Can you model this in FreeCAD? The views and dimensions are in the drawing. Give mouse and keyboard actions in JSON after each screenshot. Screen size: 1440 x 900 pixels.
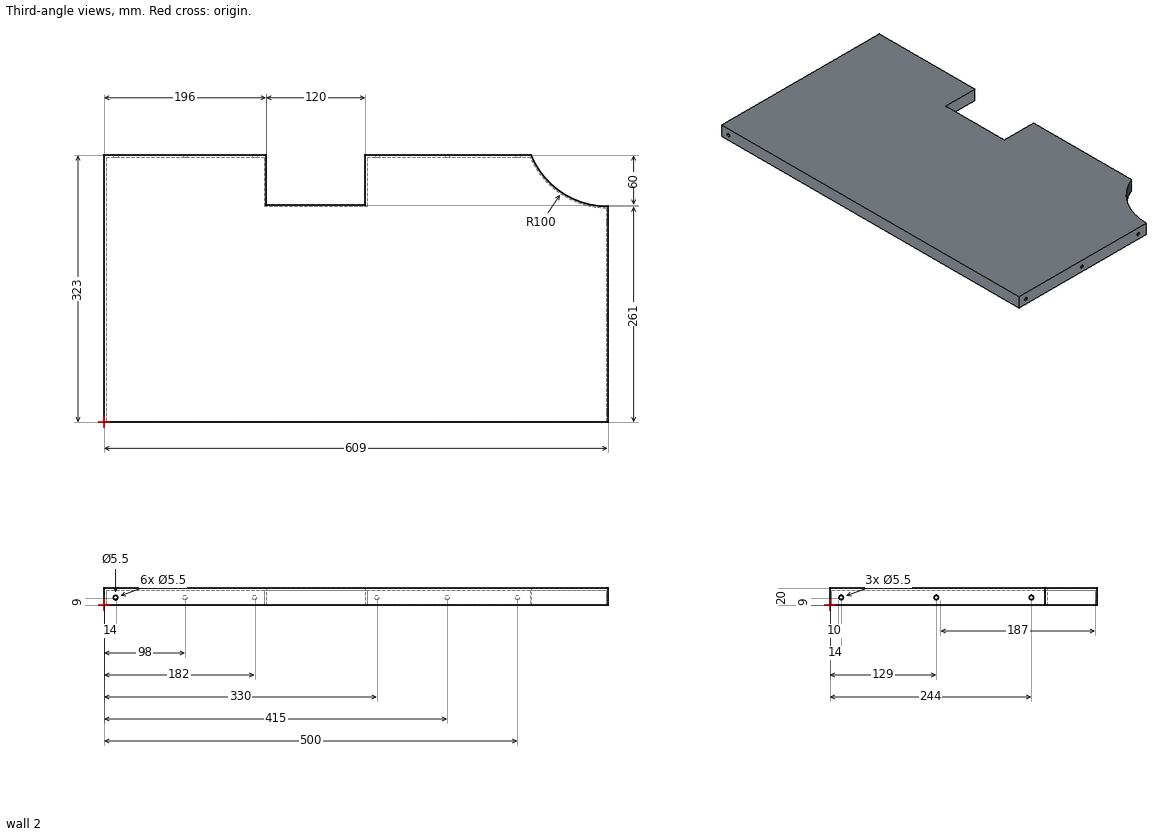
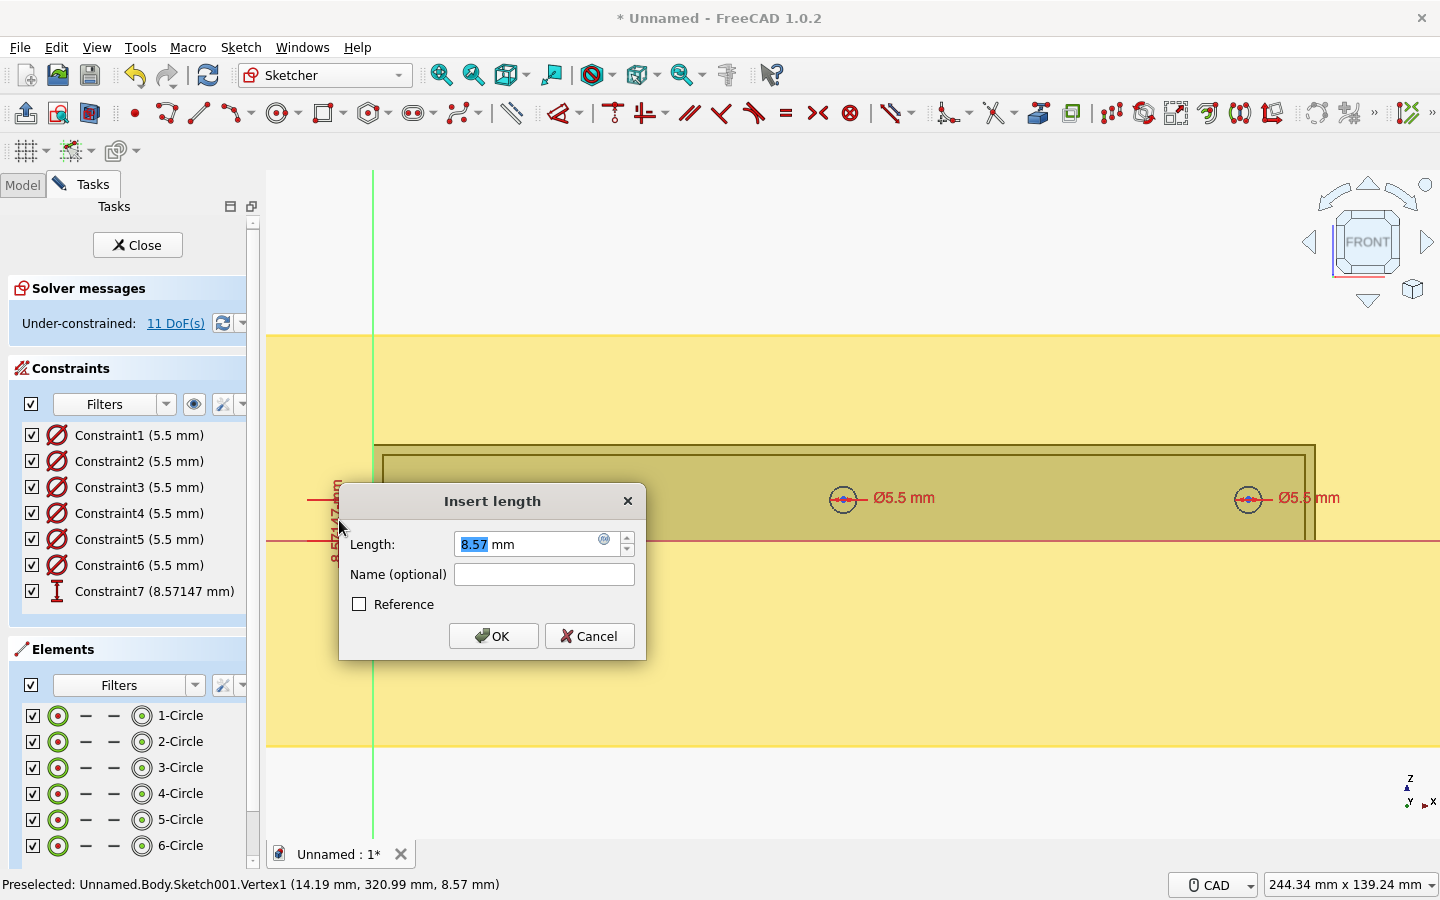
{"action": "type", "text": "9"}
{"action": "key", "text": "Return"}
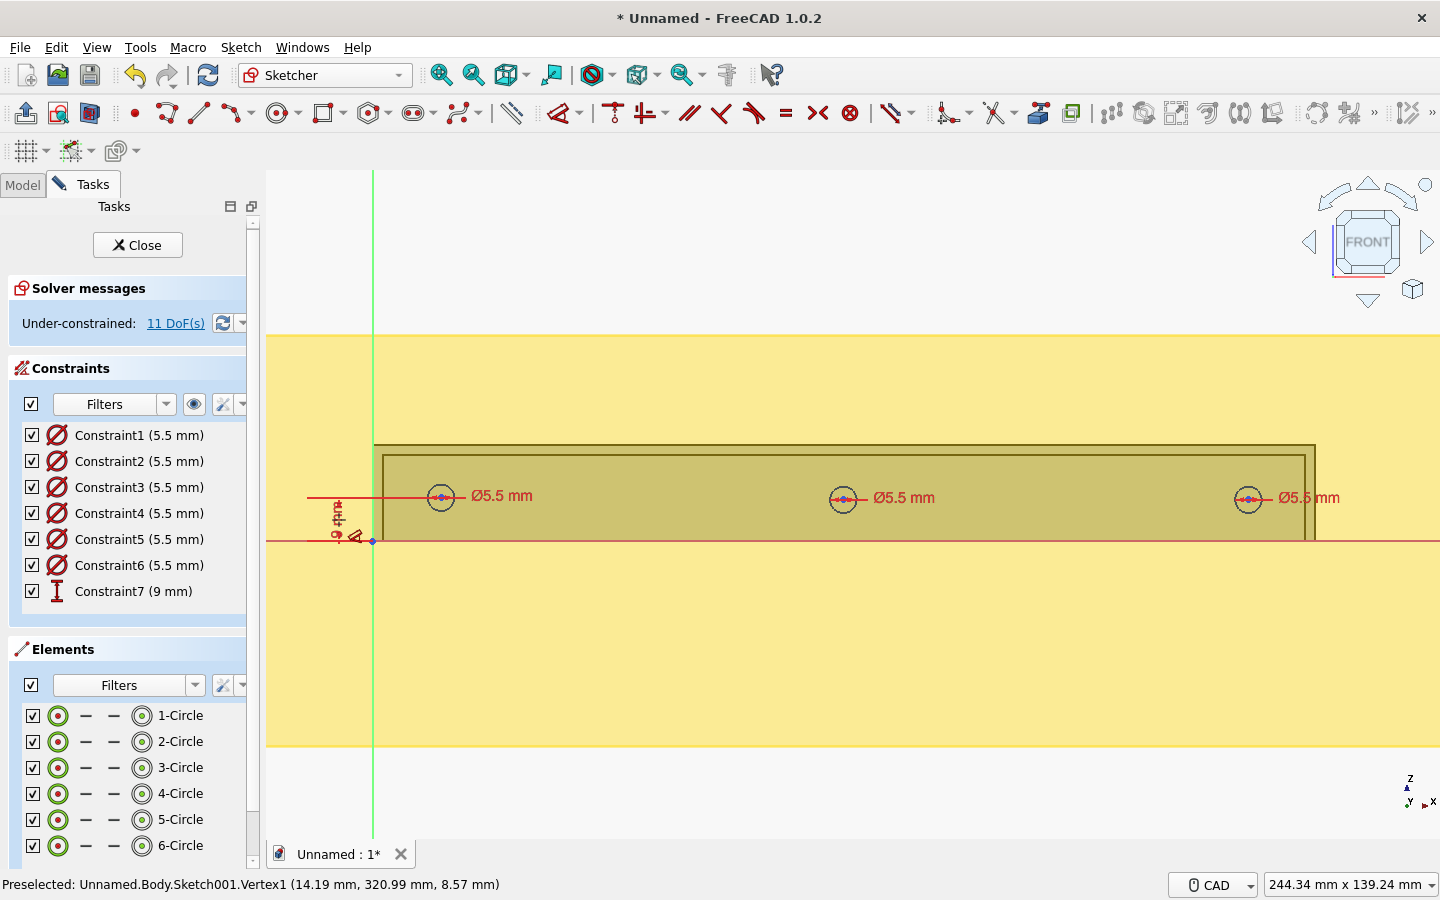
{"action": "left_click", "coordinate": [1248, 500]}
{"action": "left_click", "coordinate": [339, 506]}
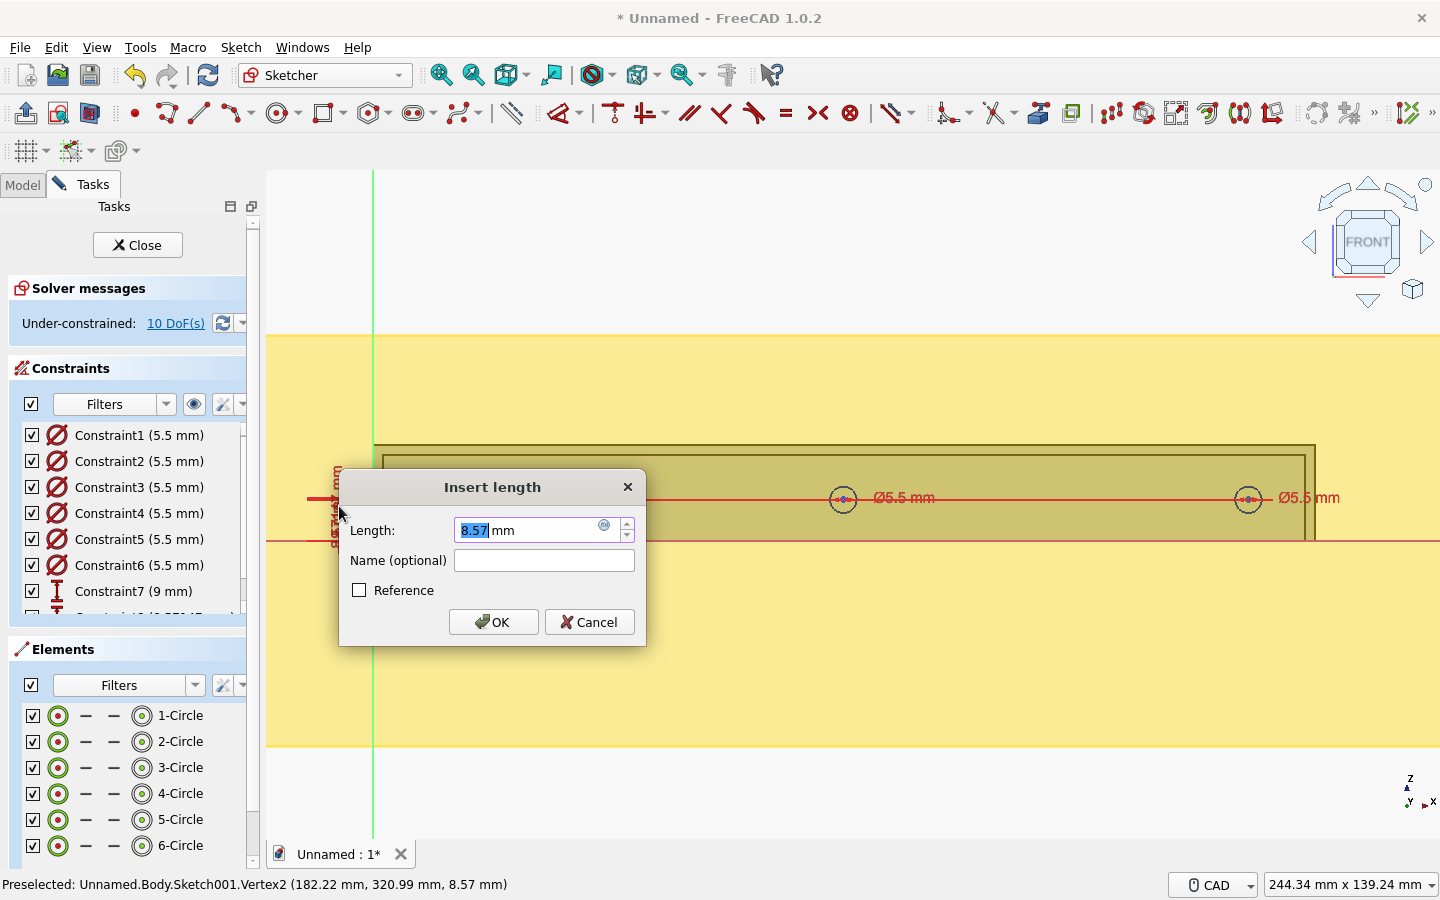
{"action": "type", "text": "9"}
{"action": "key", "text": "Return"}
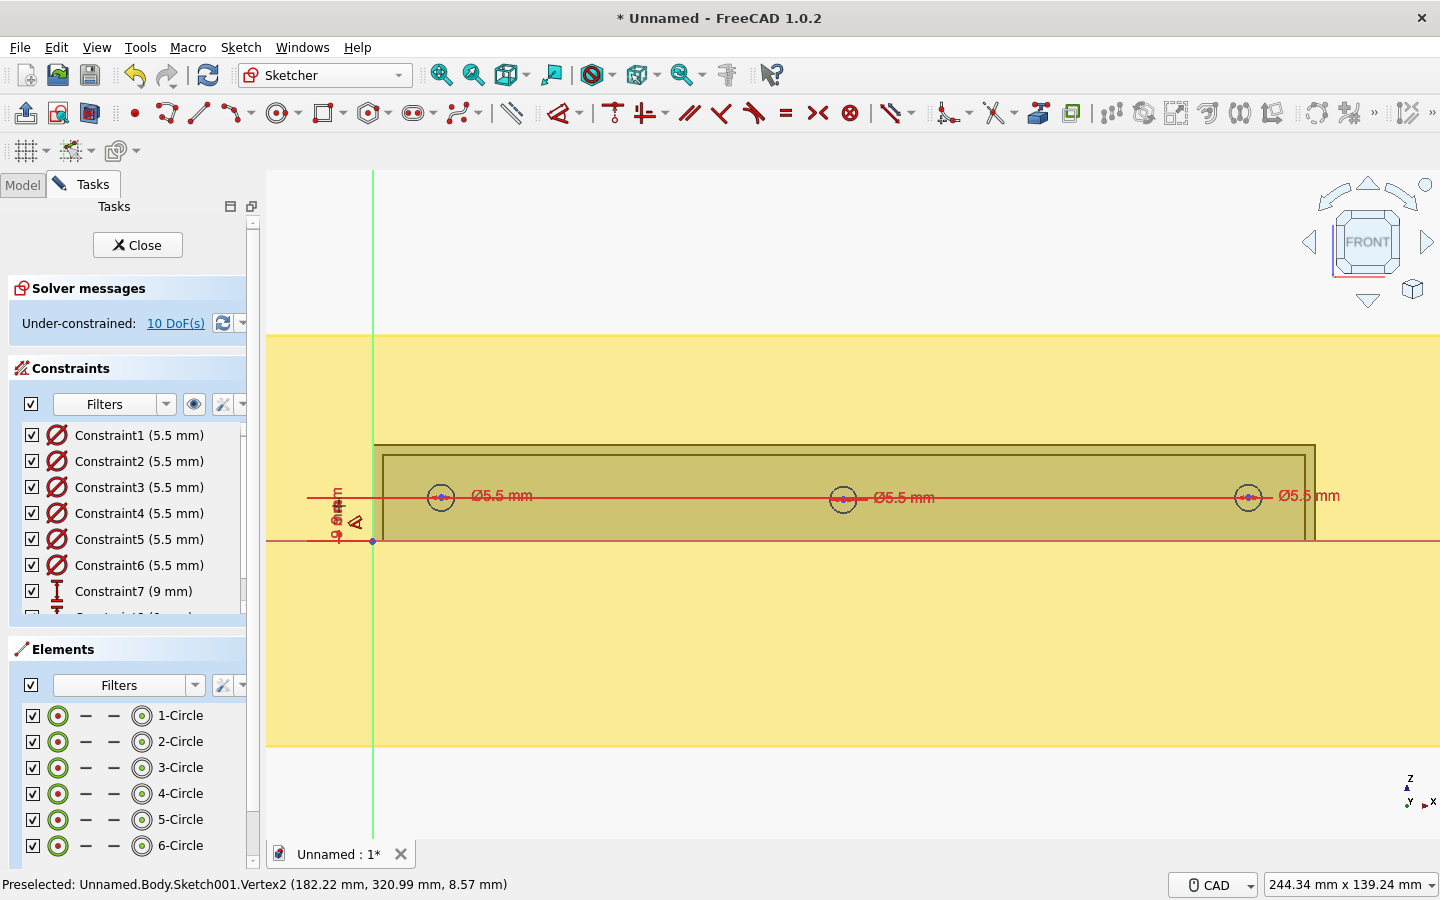
{"action": "left_click", "coordinate": [843, 500]}
{"action": "left_click", "coordinate": [877, 520]}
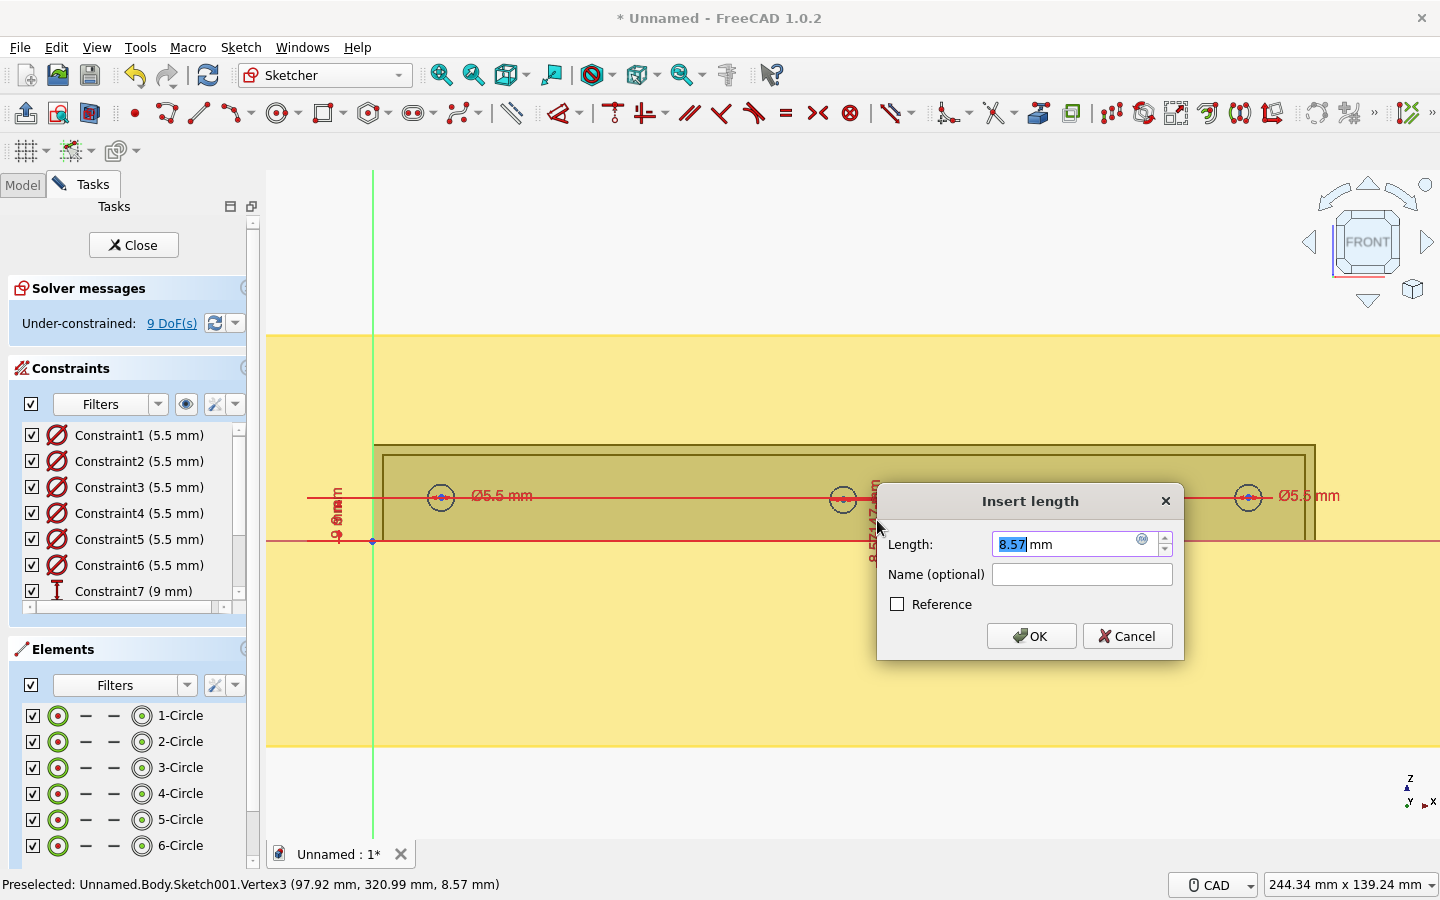
{"action": "type", "text": "9"}
{"action": "key", "text": "Return"}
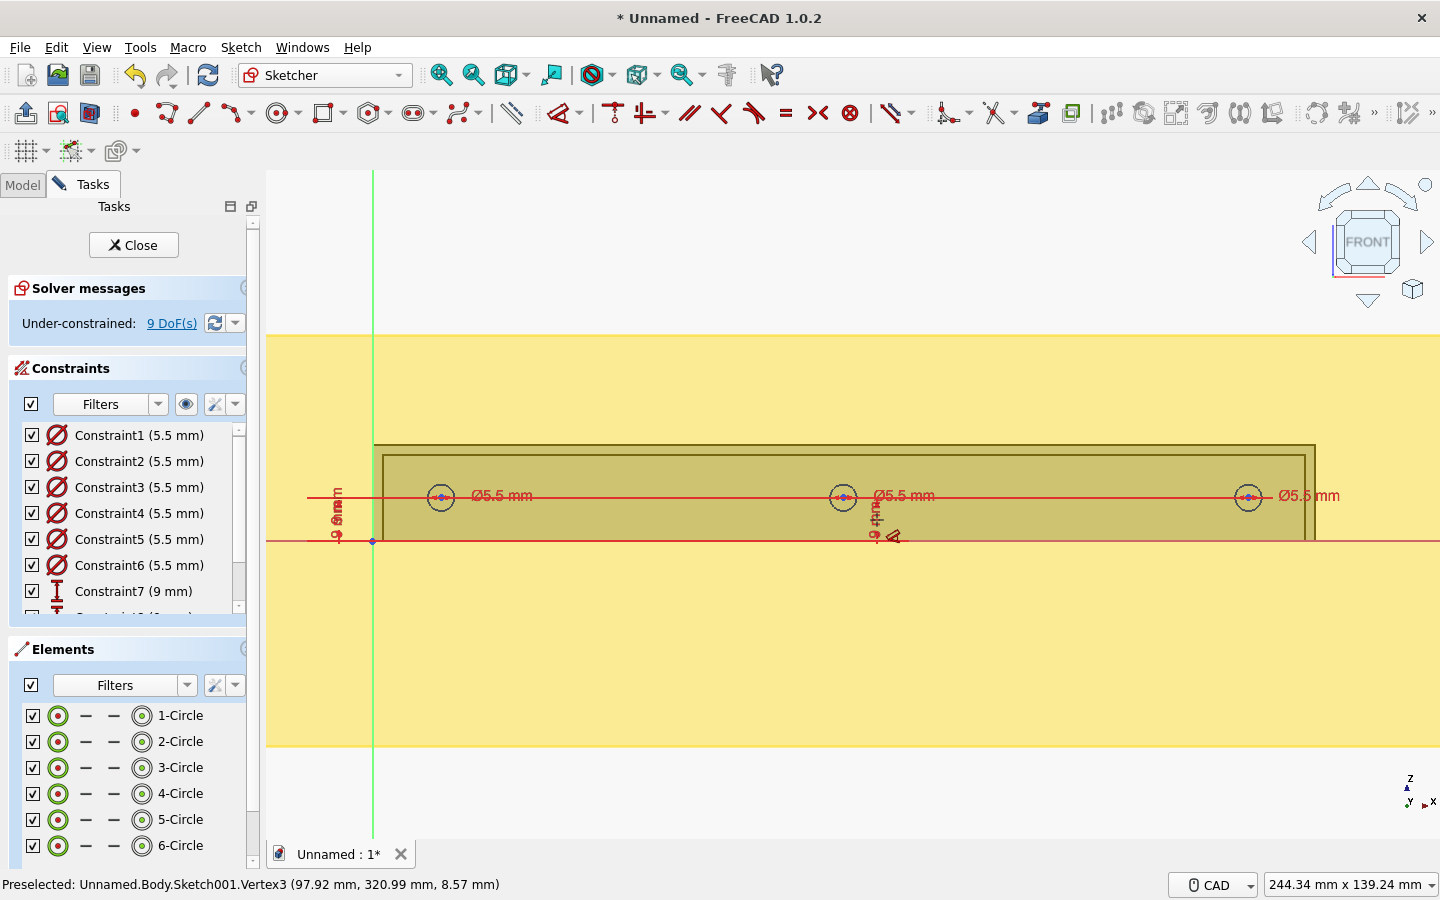
{"action": "scroll", "coordinate": [441, 501], "scroll_direction": "down", "scroll_amount": 6}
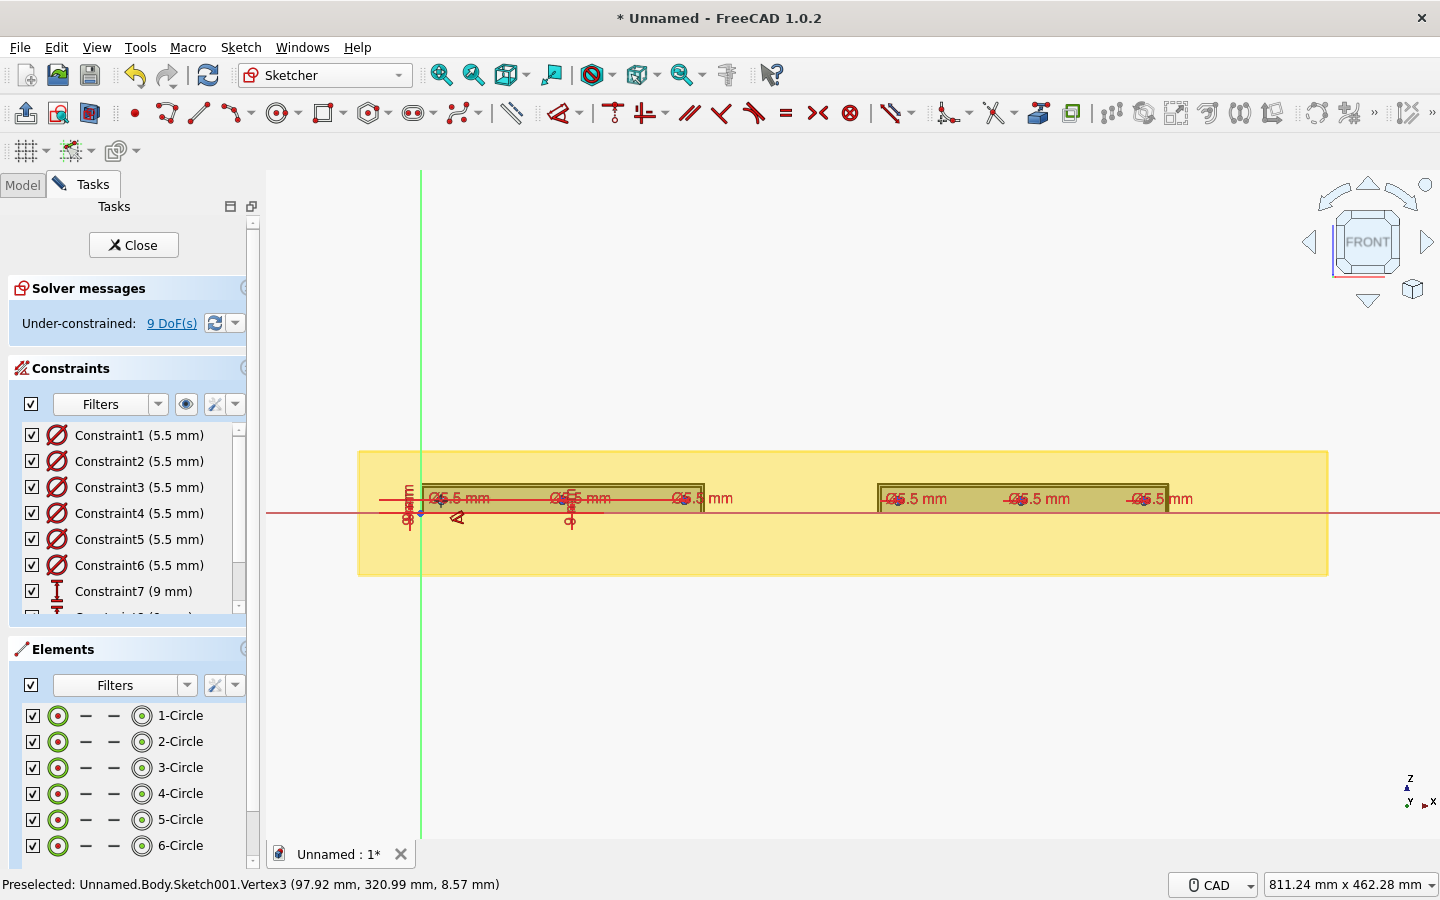
{"action": "scroll", "coordinate": [898, 501], "scroll_direction": "up", "scroll_amount": 6}